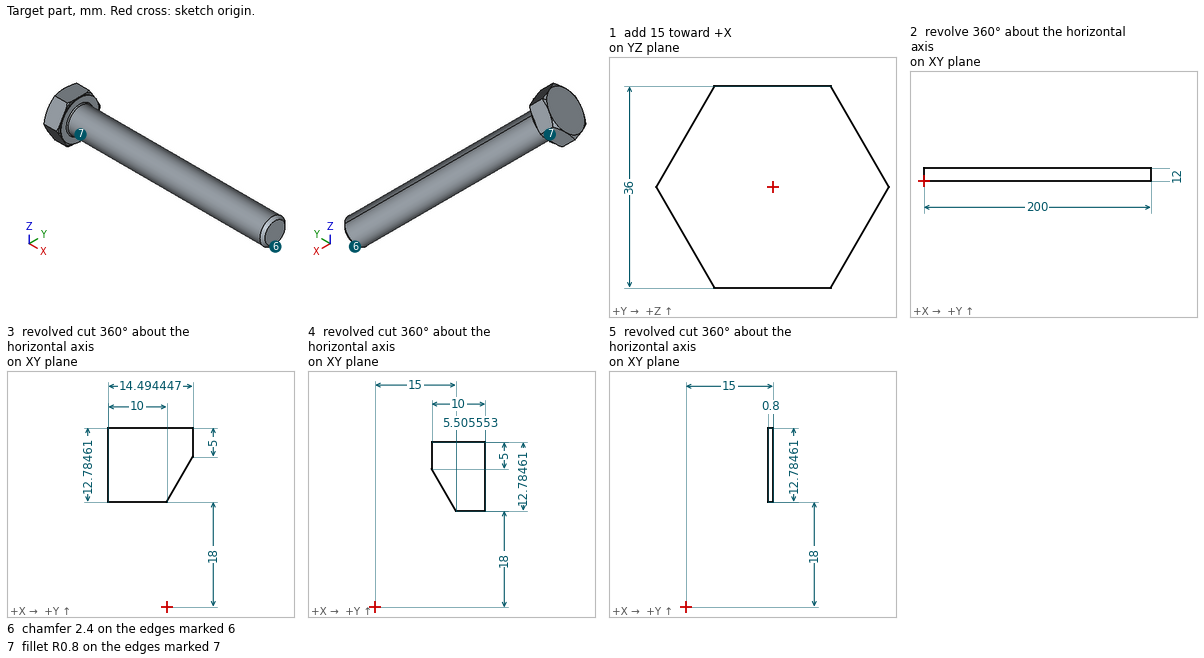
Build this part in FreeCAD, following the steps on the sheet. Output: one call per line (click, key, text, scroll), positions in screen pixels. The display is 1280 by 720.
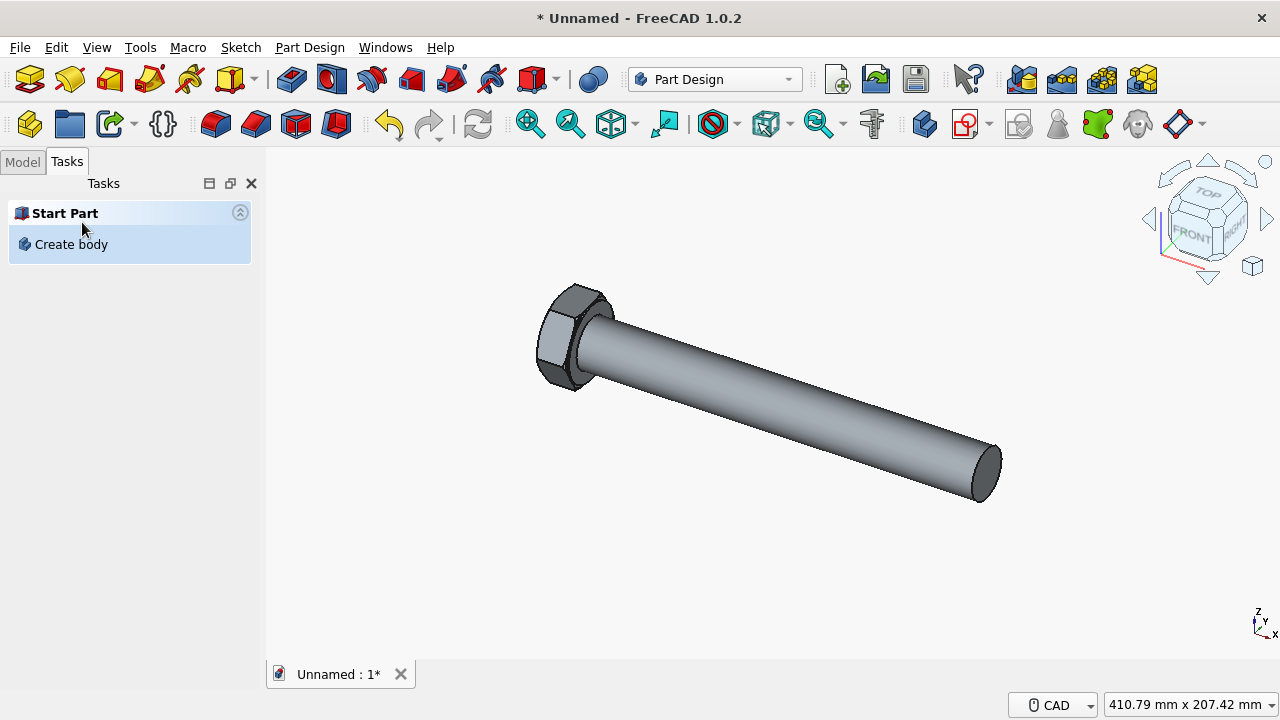
click(972, 488)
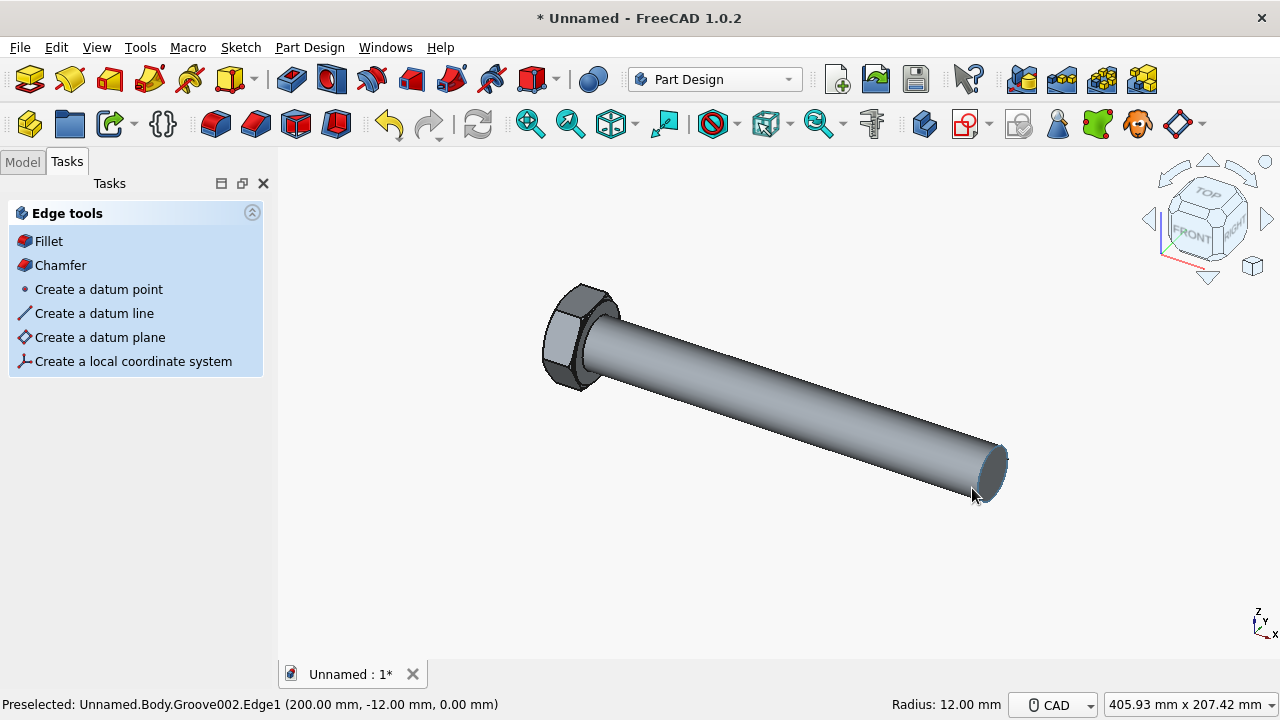
click(256, 124)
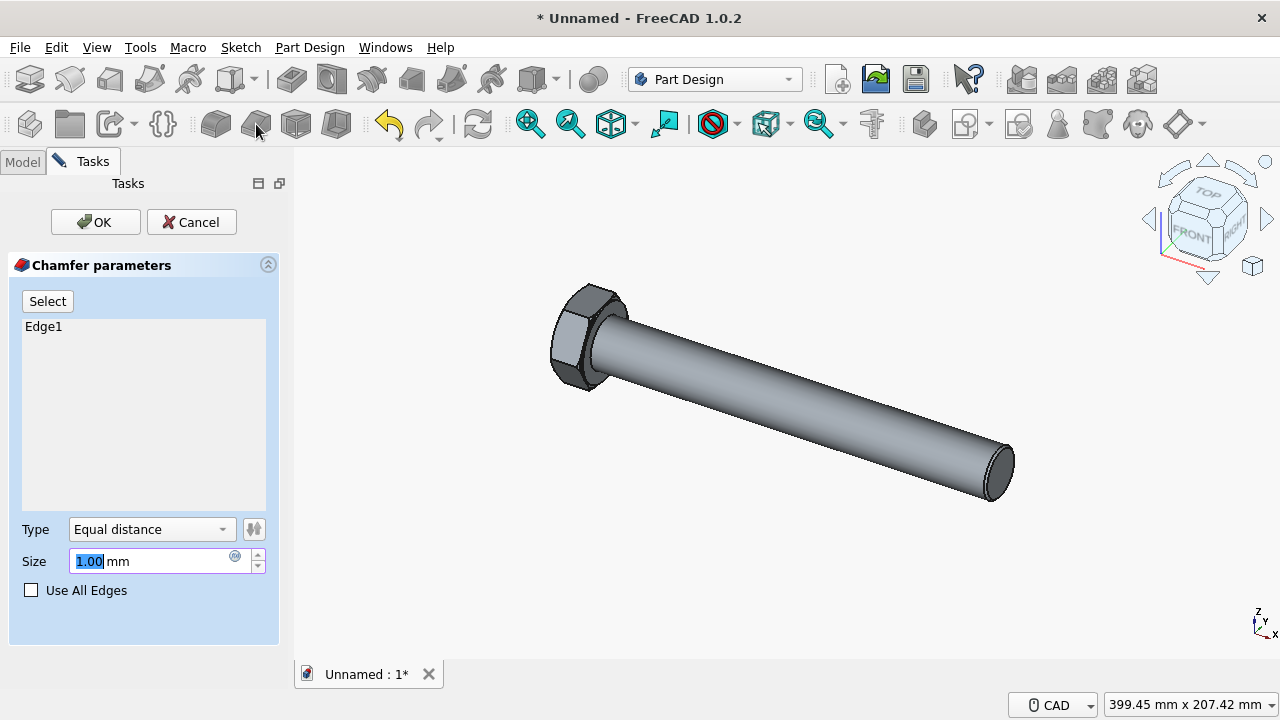
text(2.4)
key(Tab)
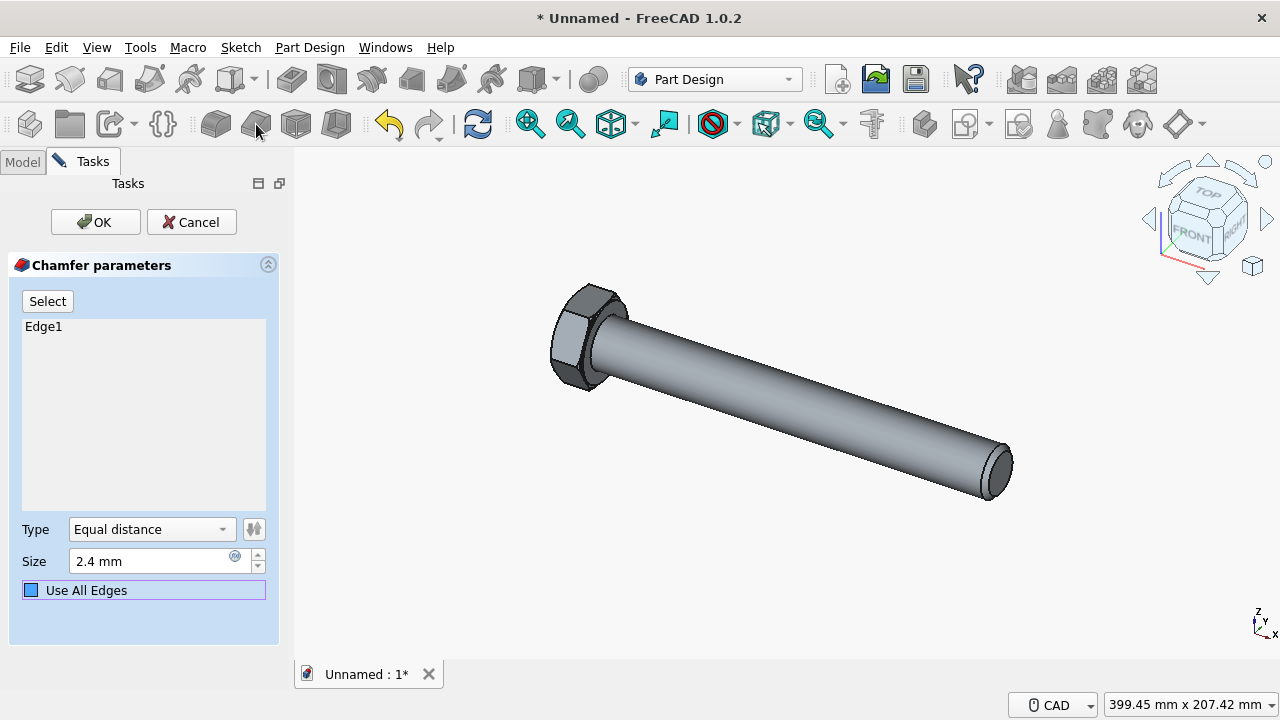
click(96, 222)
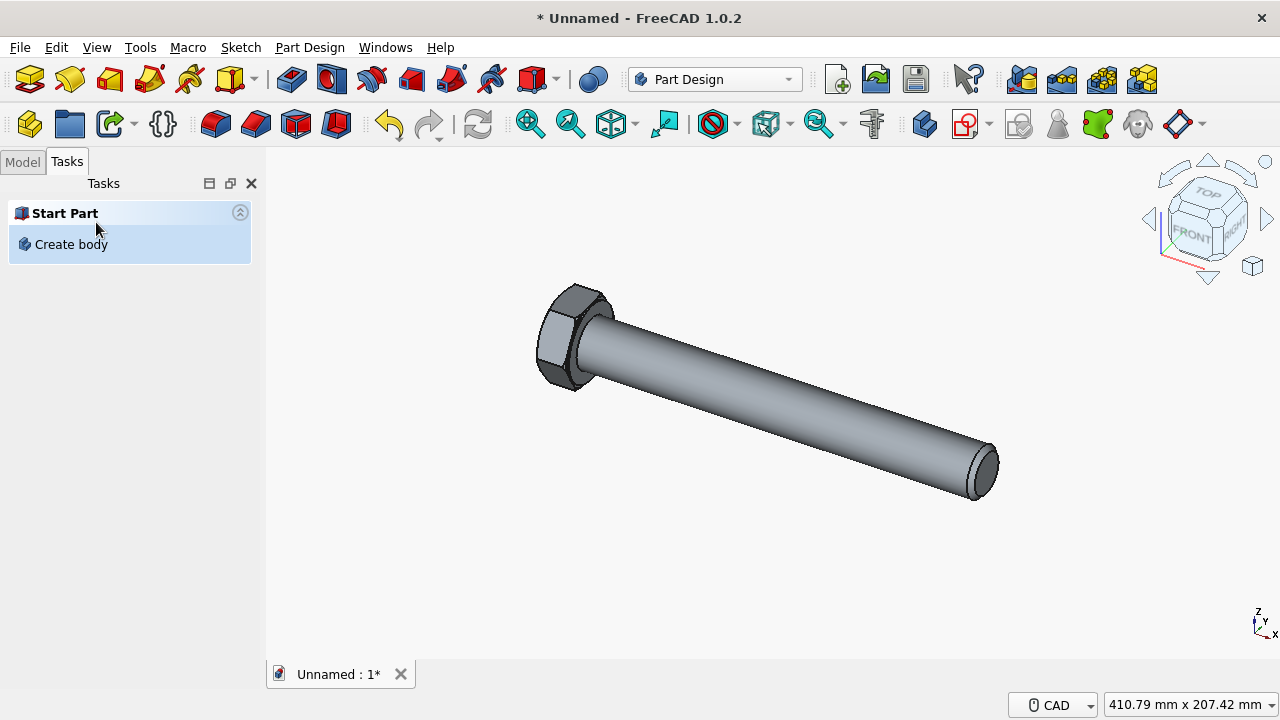
key(0)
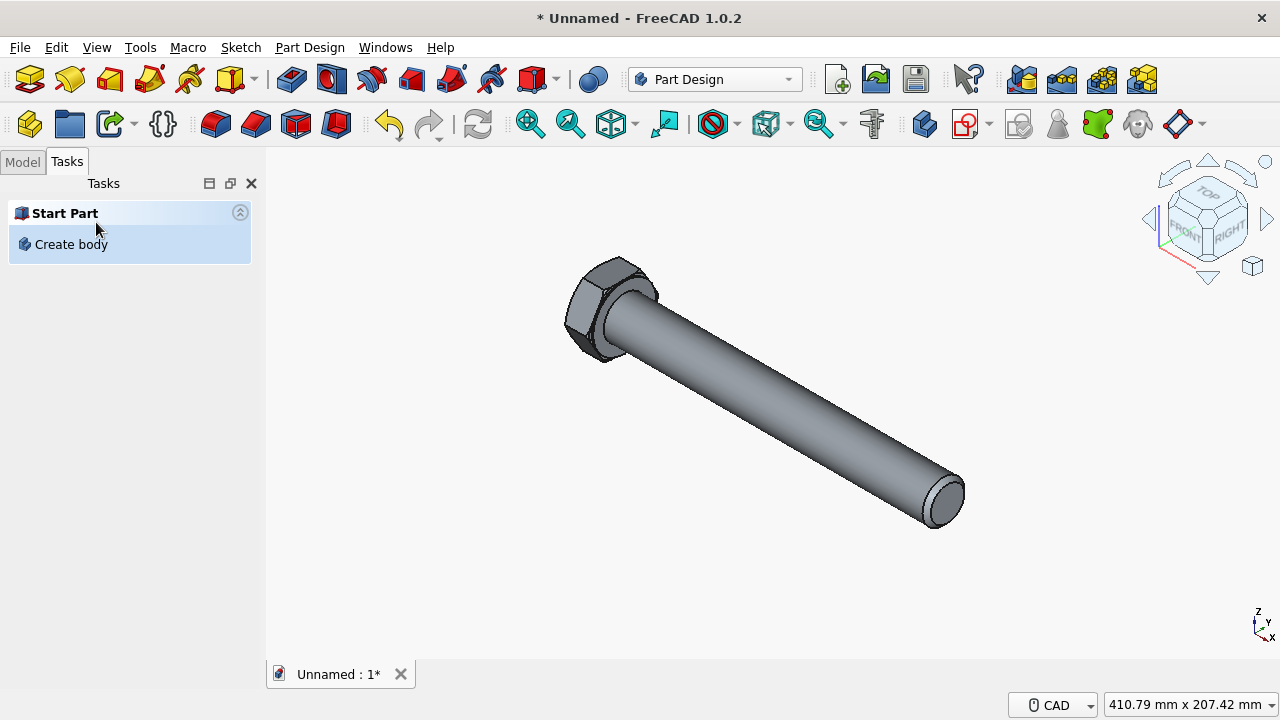
key(2)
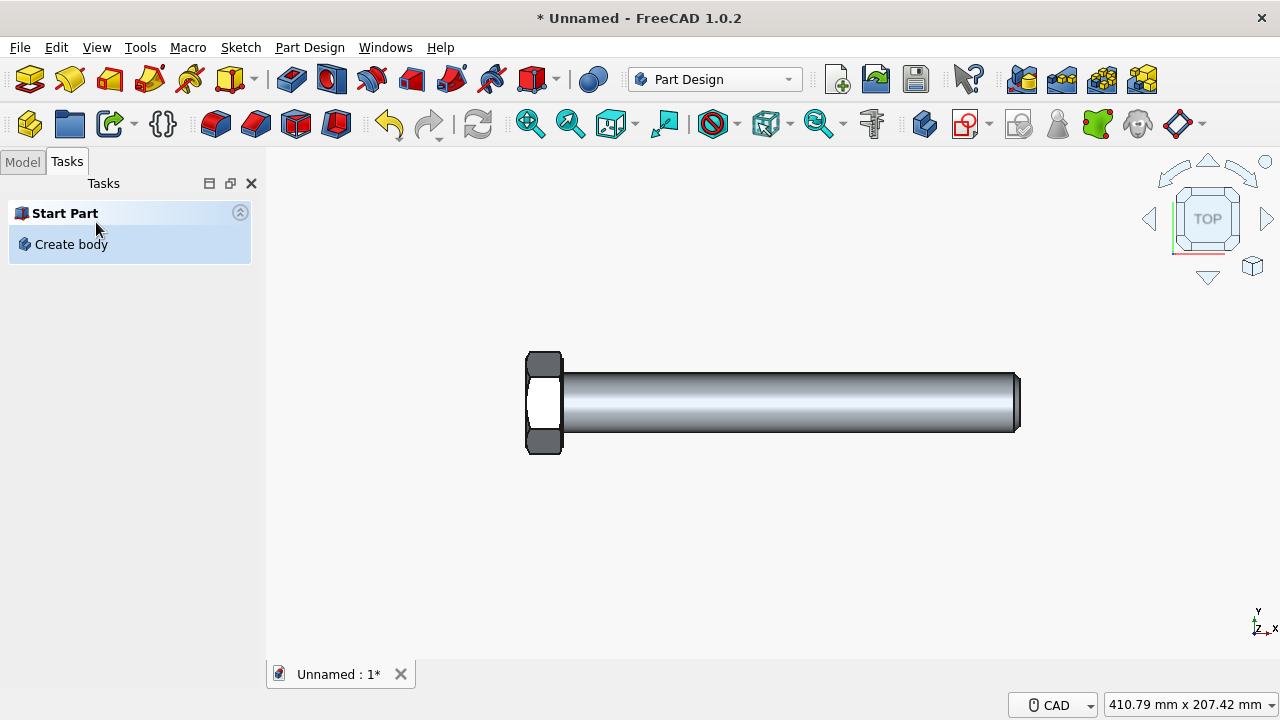
key(1)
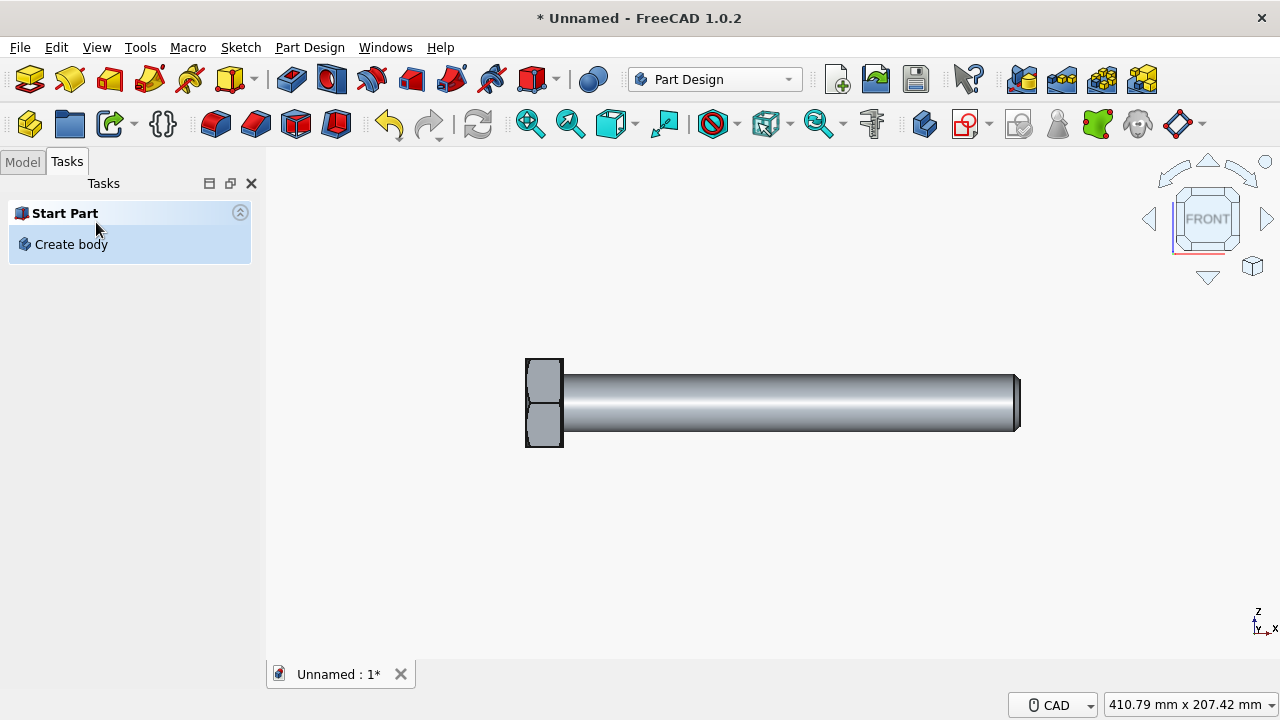
key(3)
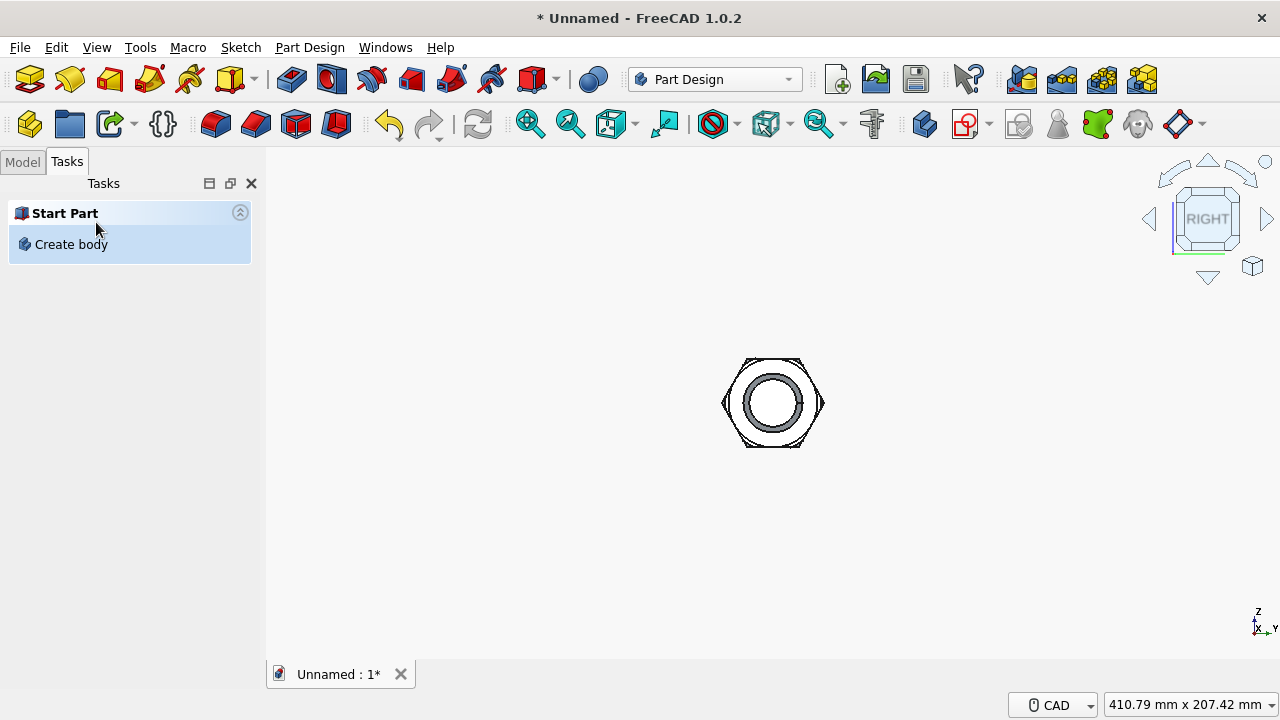
click(532, 124)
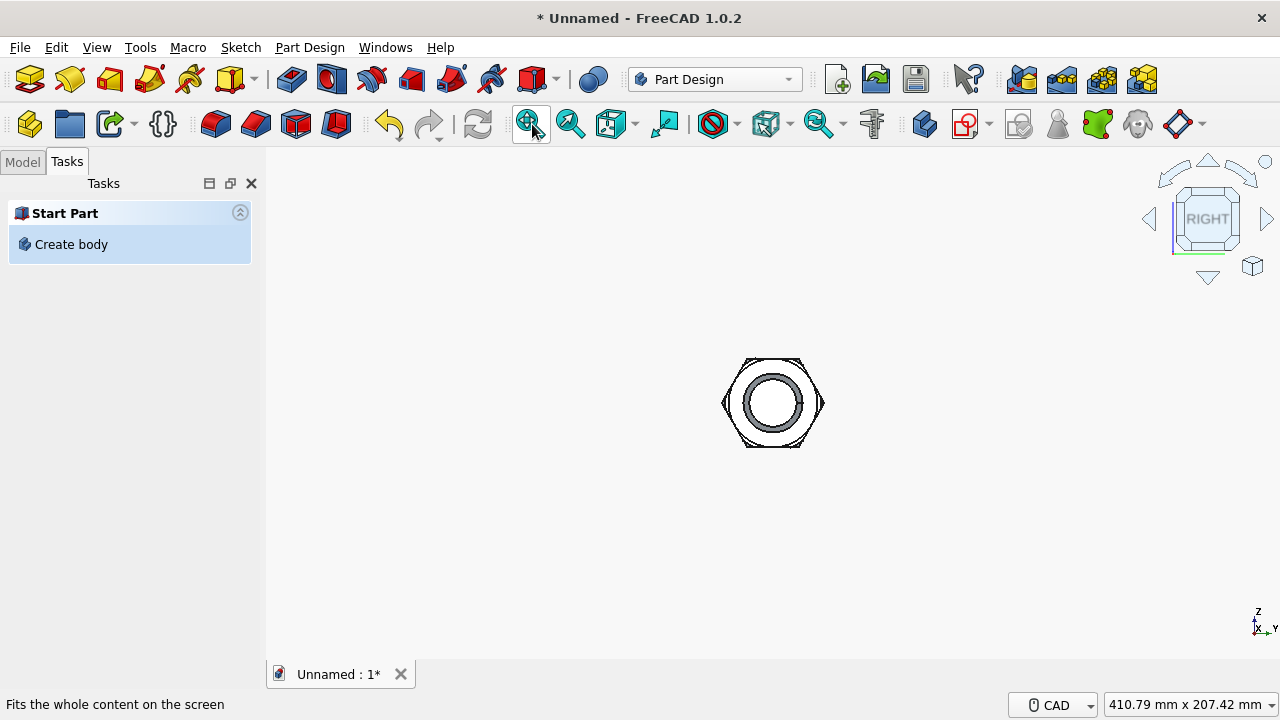
key(5)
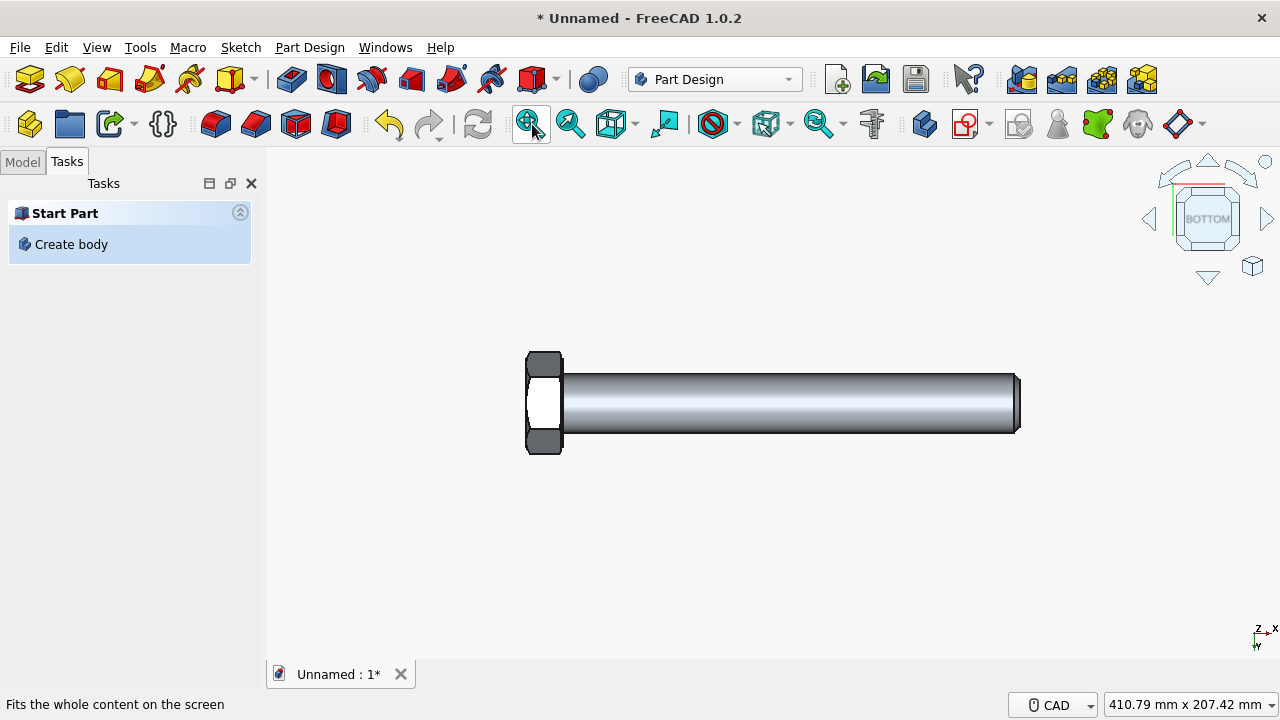
key(4)